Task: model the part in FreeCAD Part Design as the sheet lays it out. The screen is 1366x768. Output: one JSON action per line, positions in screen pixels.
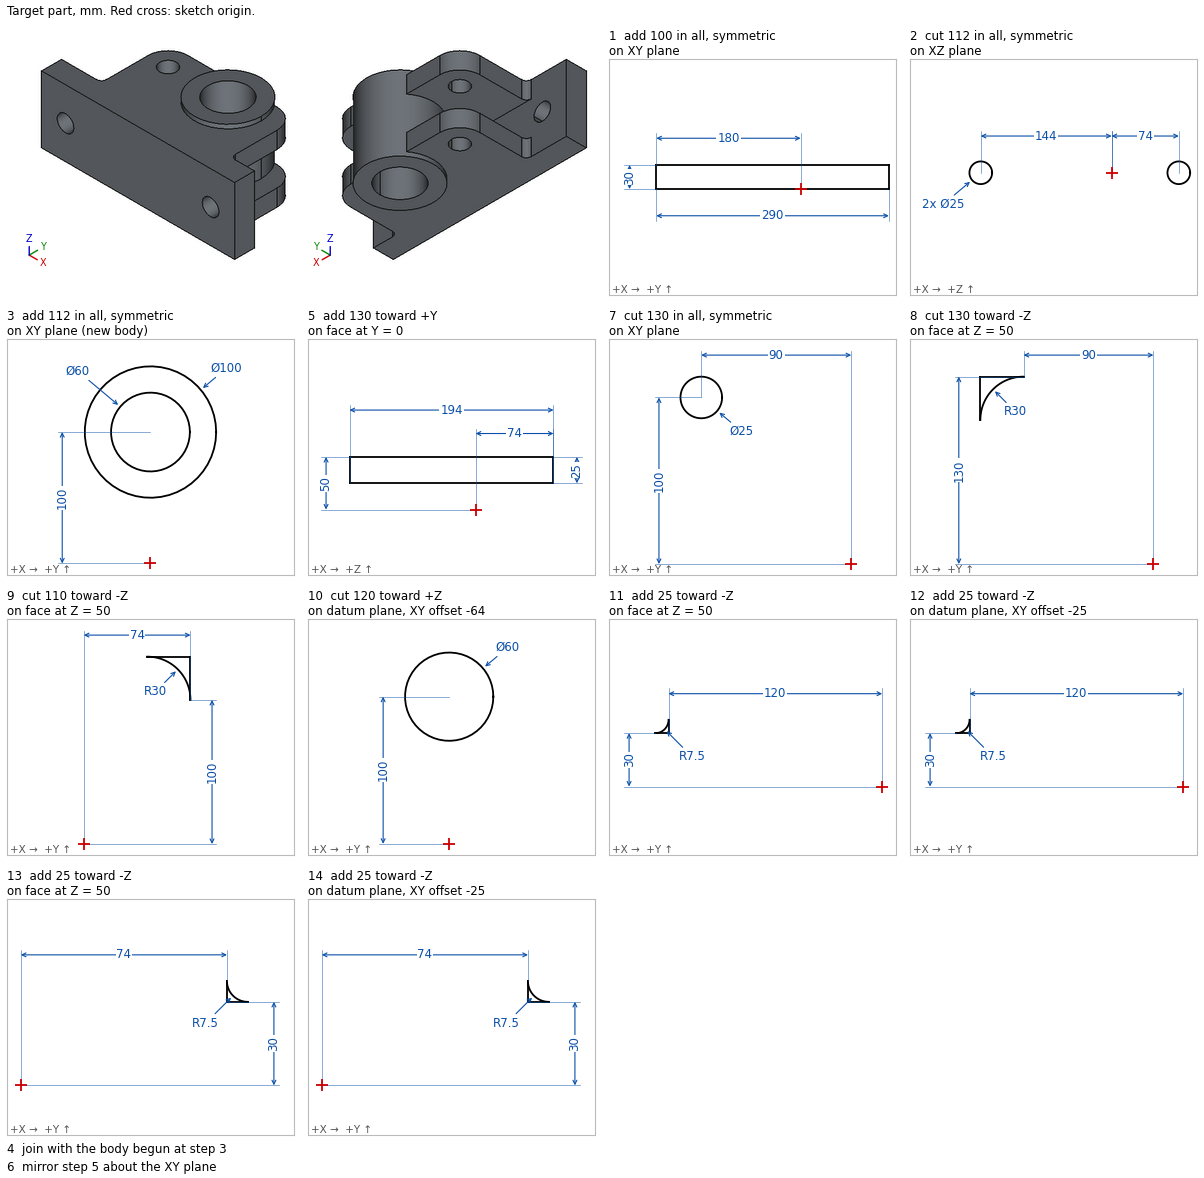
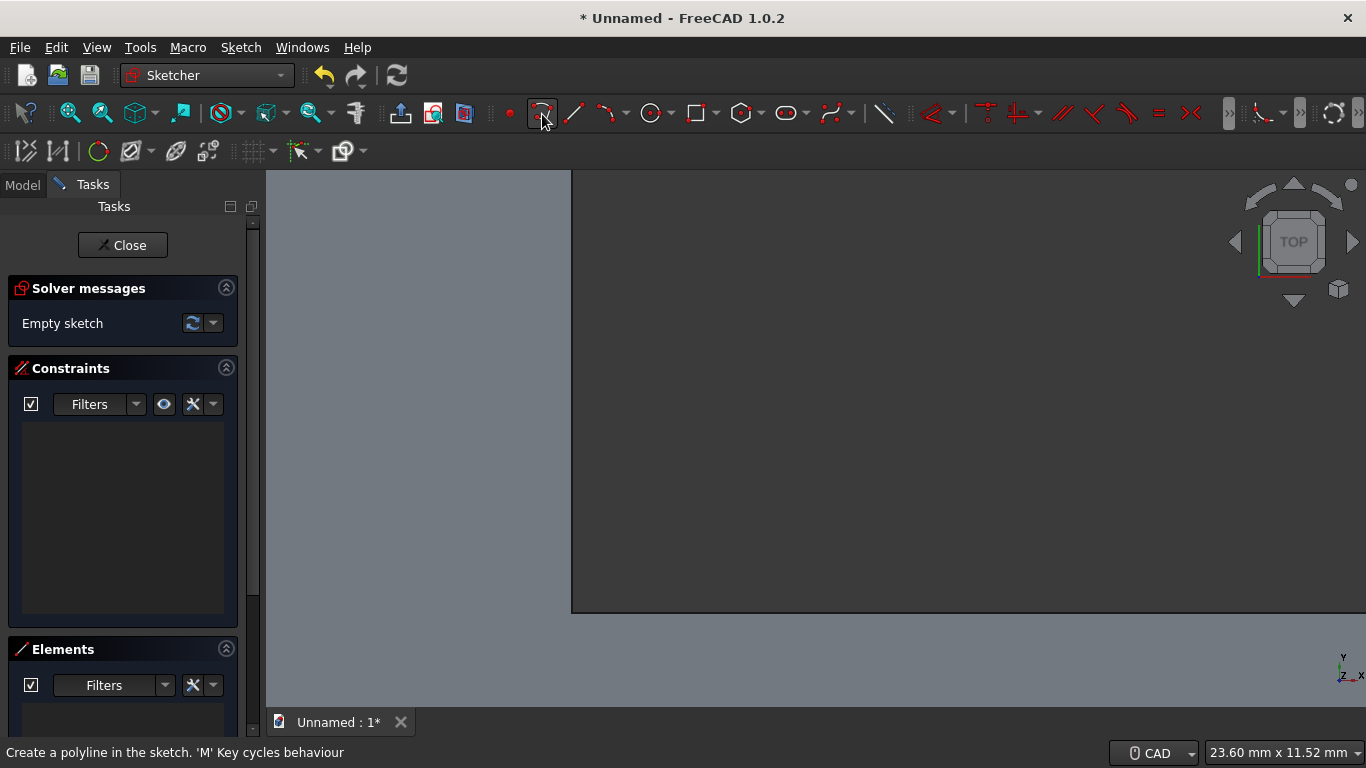
{"action": "left_click", "coordinate": [572, 263]}
{"action": "left_click", "coordinate": [572, 613]}
{"action": "left_click", "coordinate": [922, 613]}
{"action": "right_click", "coordinate": [922, 613]}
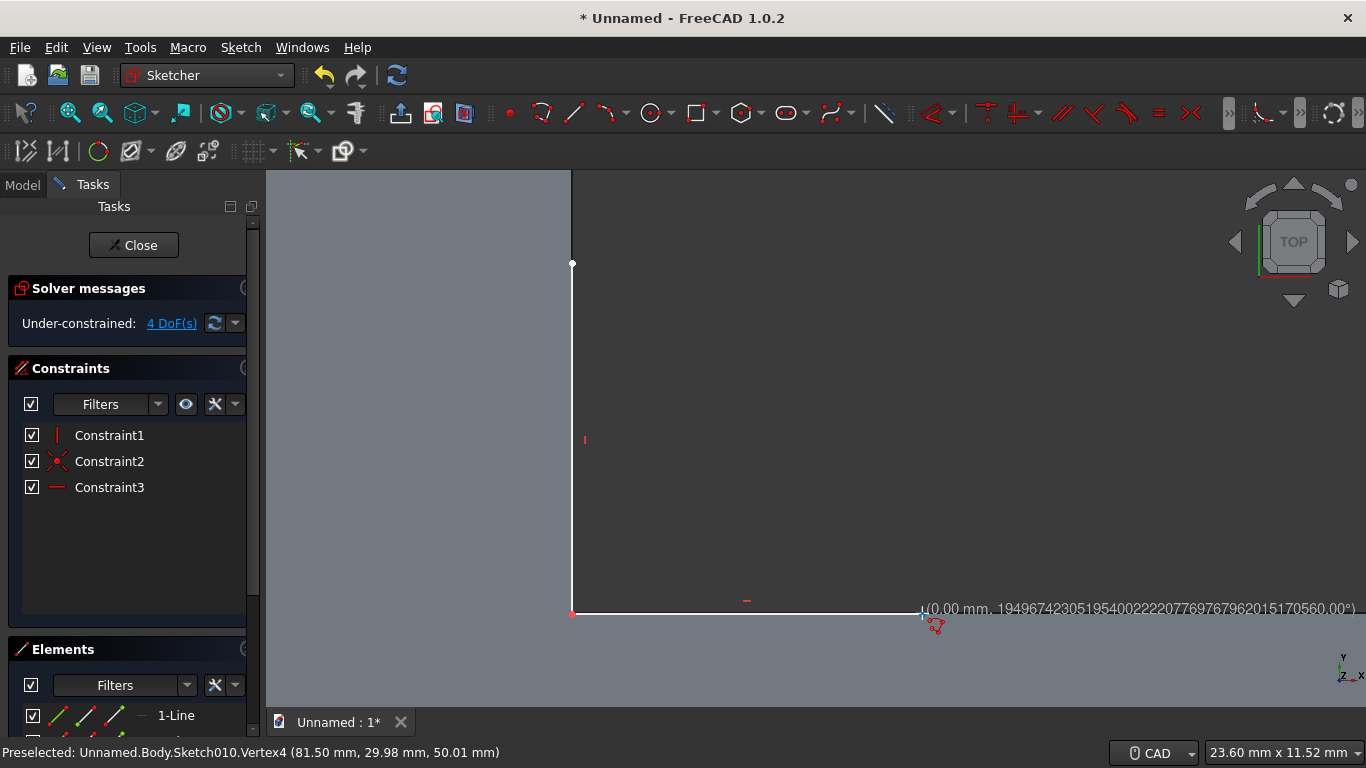
{"action": "left_click", "coordinate": [606, 114]}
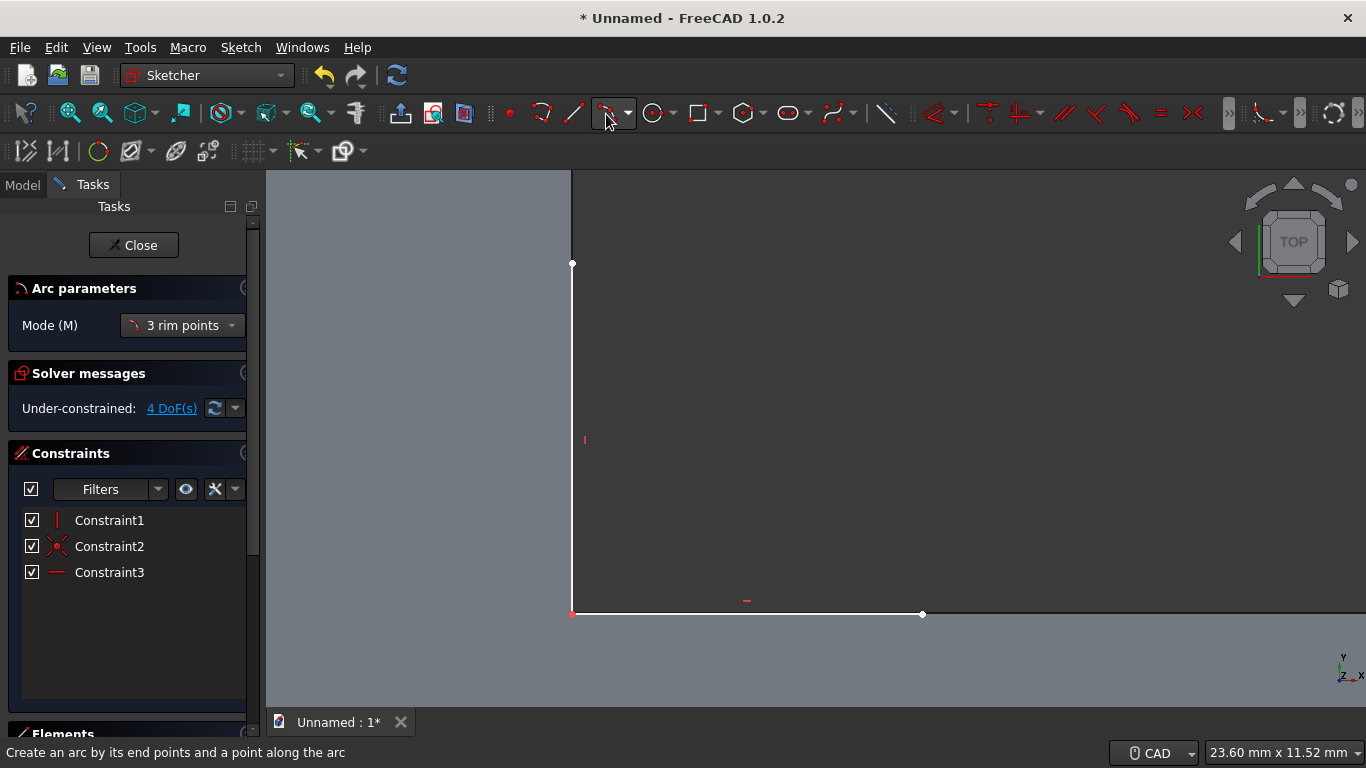
{"action": "left_click", "coordinate": [922, 614]}
{"action": "left_click", "coordinate": [572, 264]}
{"action": "left_click", "coordinate": [675, 511]}
{"action": "key", "text": "Escape"}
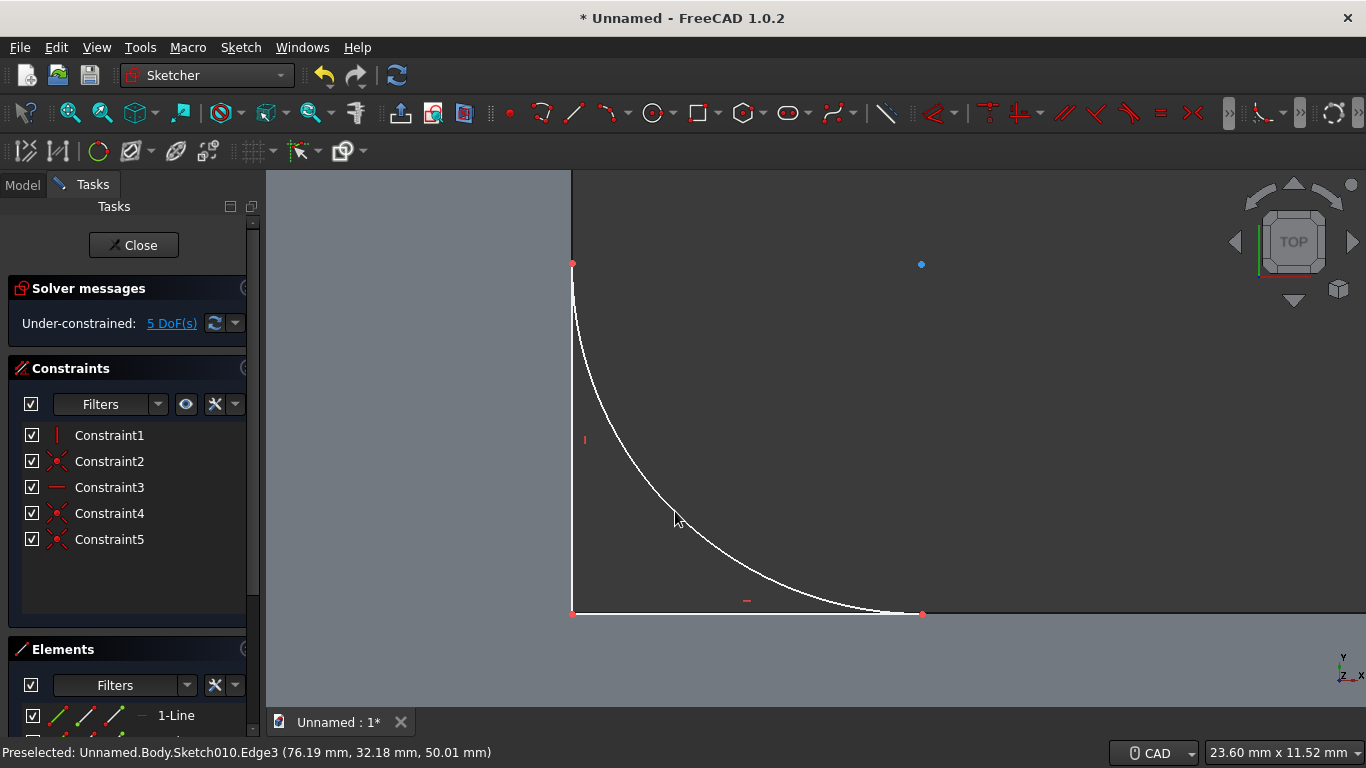
{"action": "left_click", "coordinate": [572, 369]}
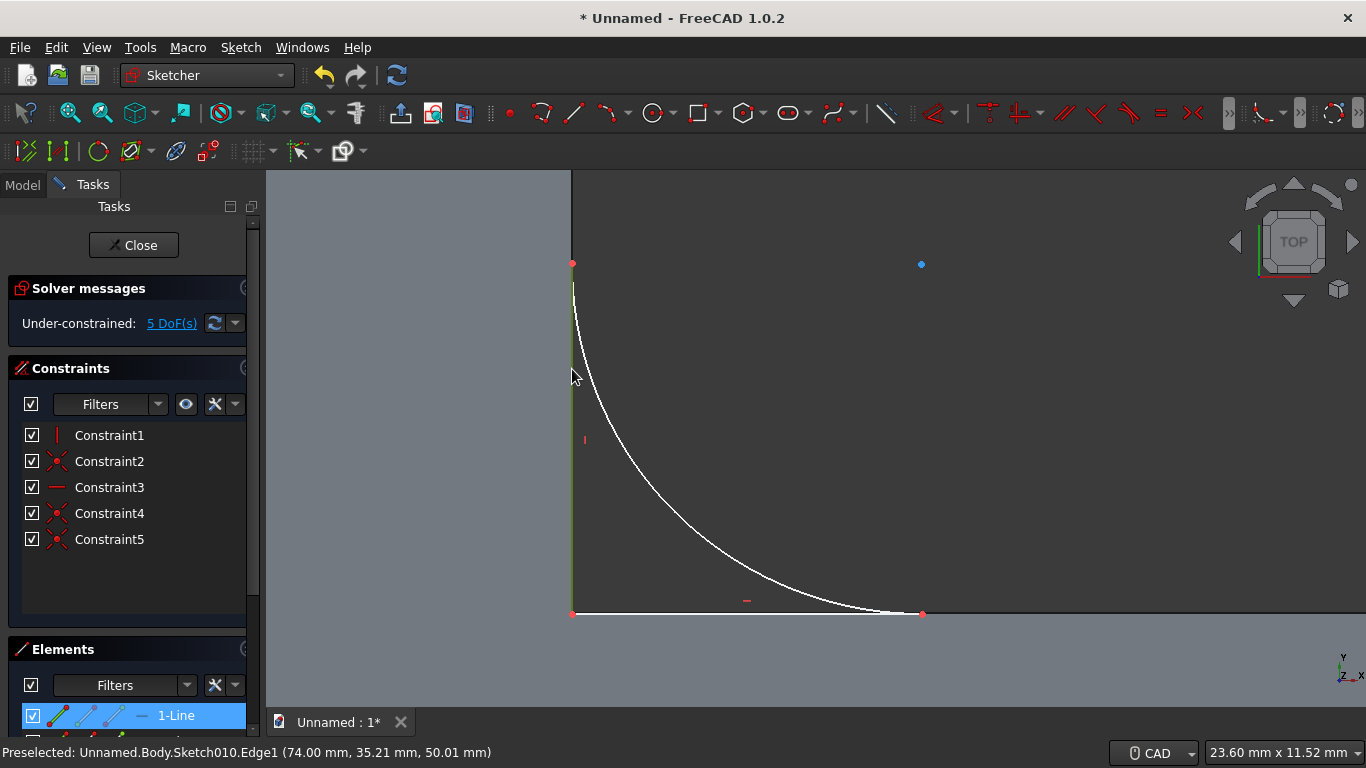
{"action": "left_click", "coordinate": [610, 423]}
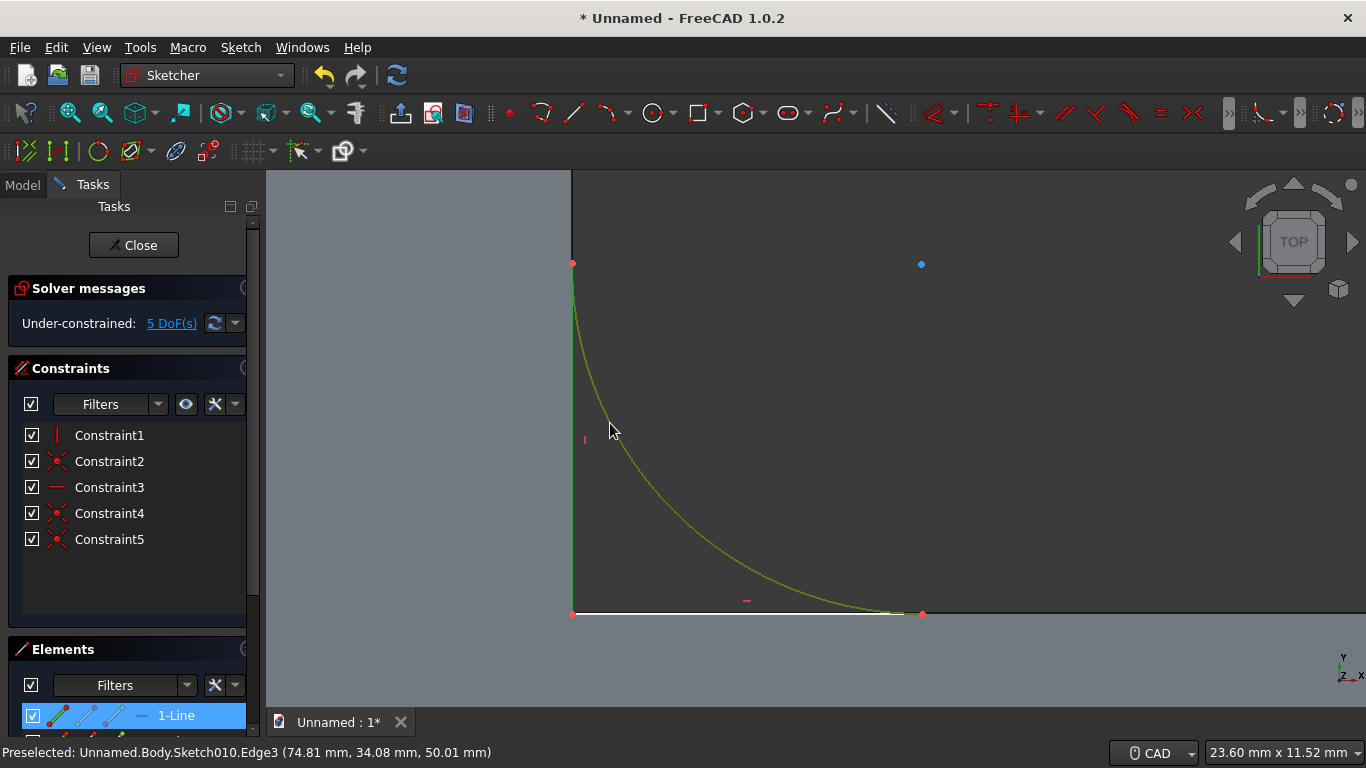
{"action": "left_click", "coordinate": [1130, 114]}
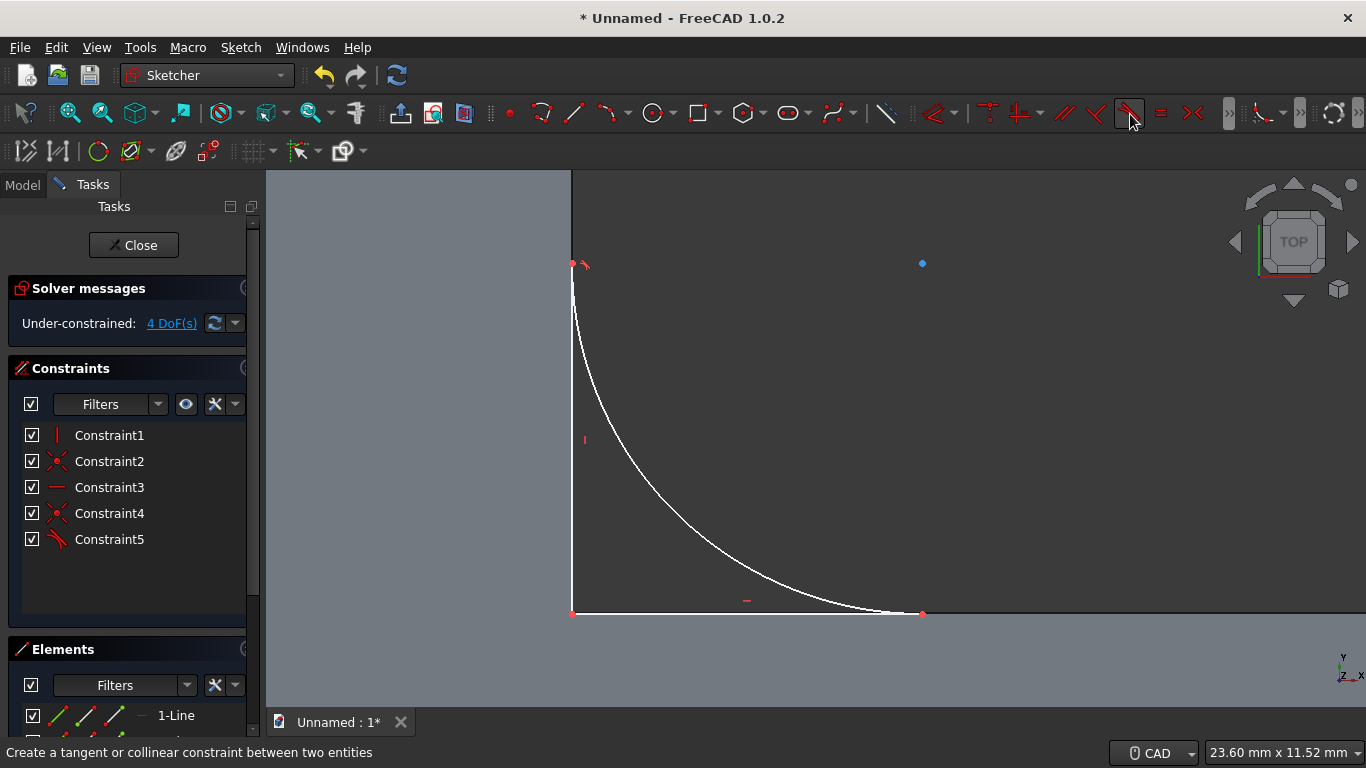
{"action": "left_click", "coordinate": [677, 614]}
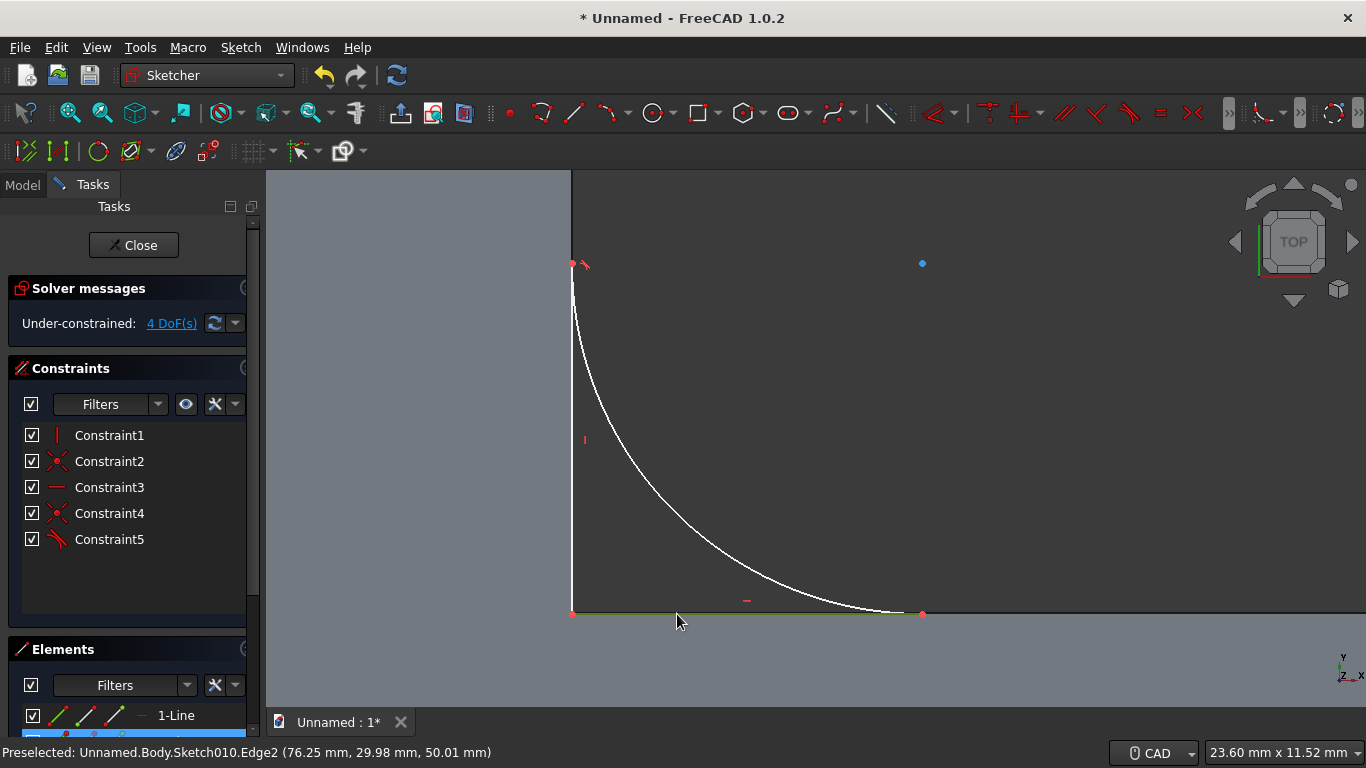
{"action": "left_click", "coordinate": [610, 423]}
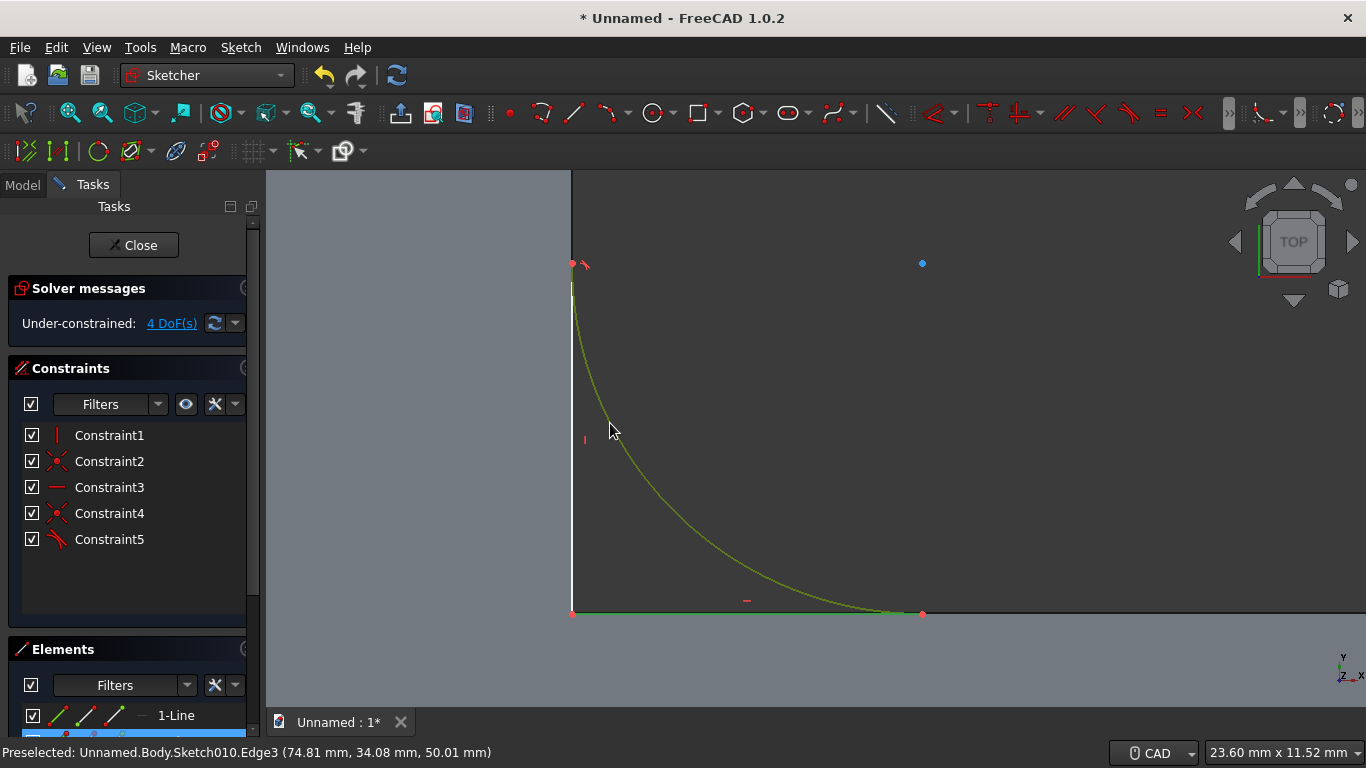
{"action": "left_click", "coordinate": [1130, 114]}